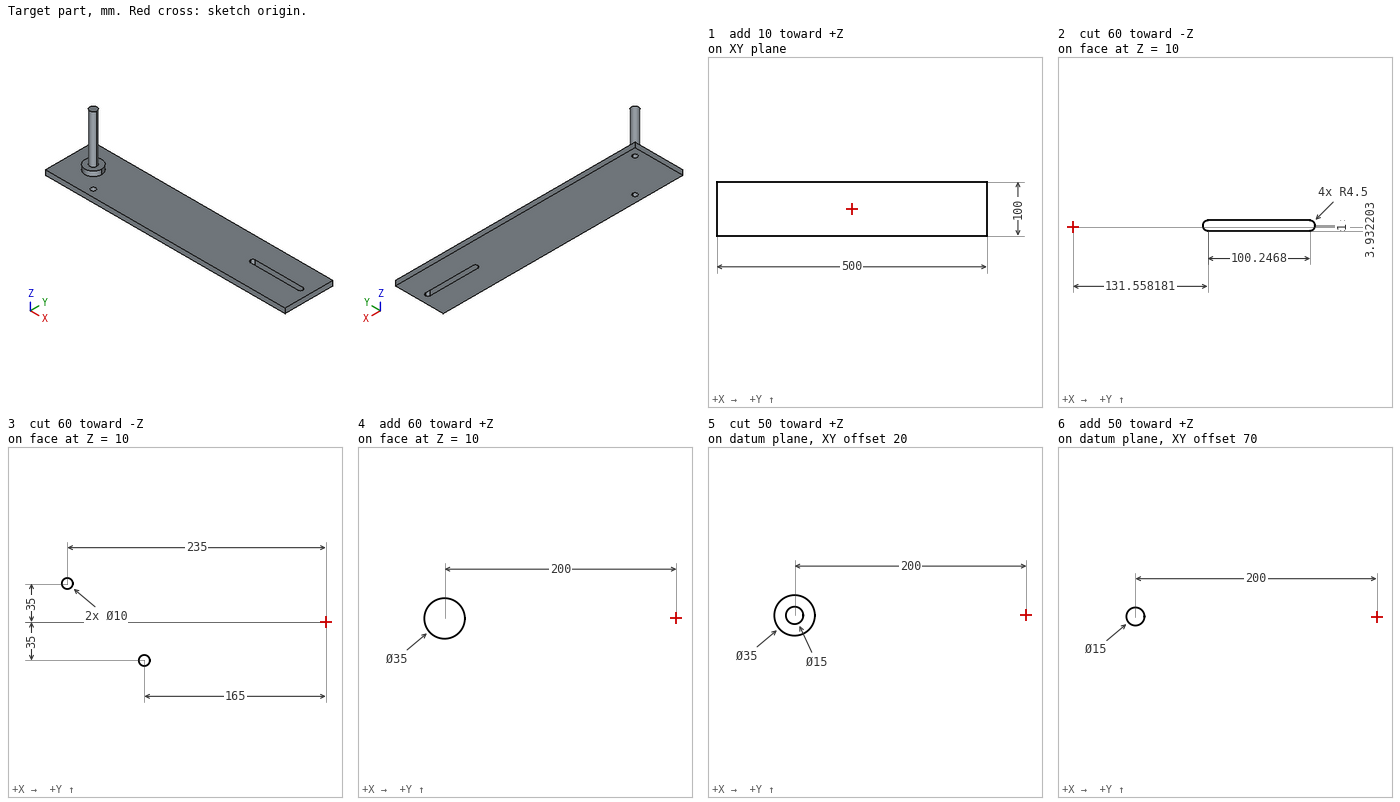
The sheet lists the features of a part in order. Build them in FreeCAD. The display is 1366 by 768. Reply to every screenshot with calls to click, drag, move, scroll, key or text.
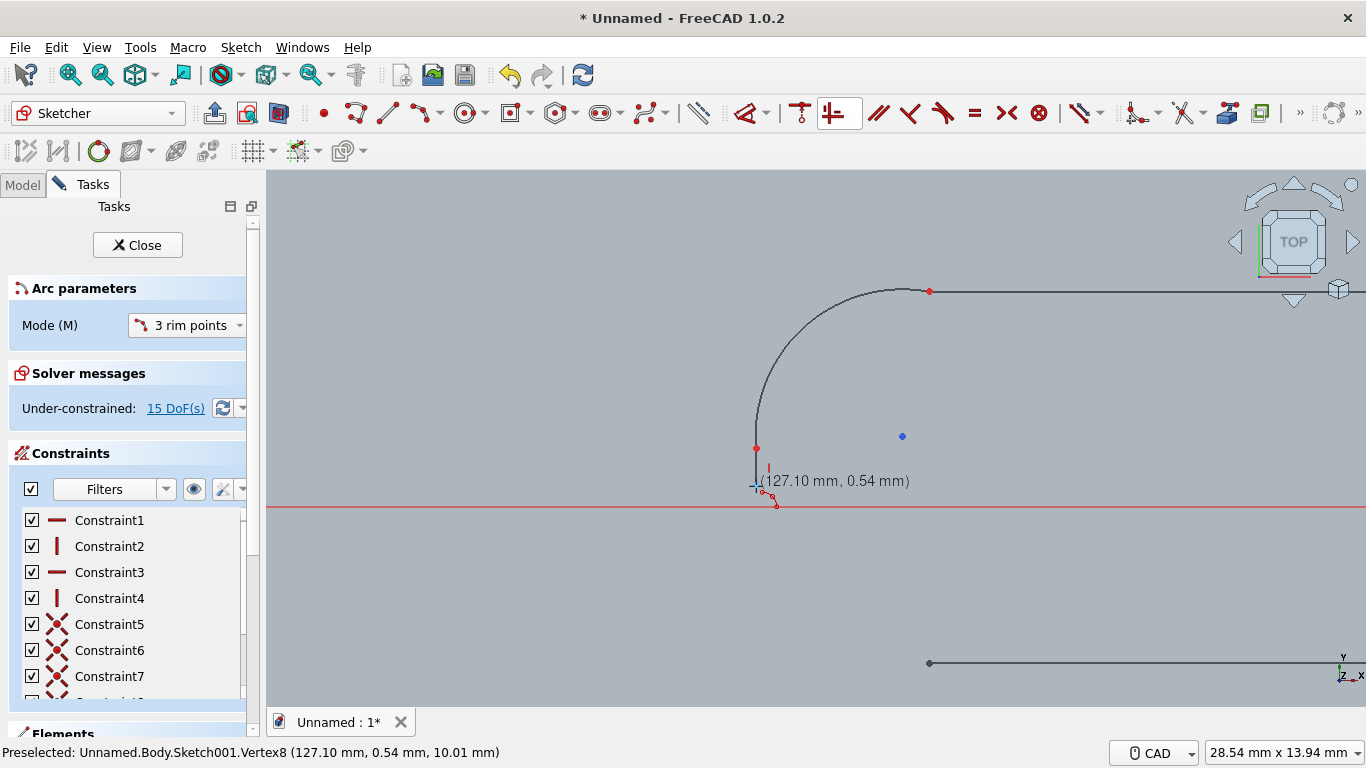
scroll(774, 436, down, 13)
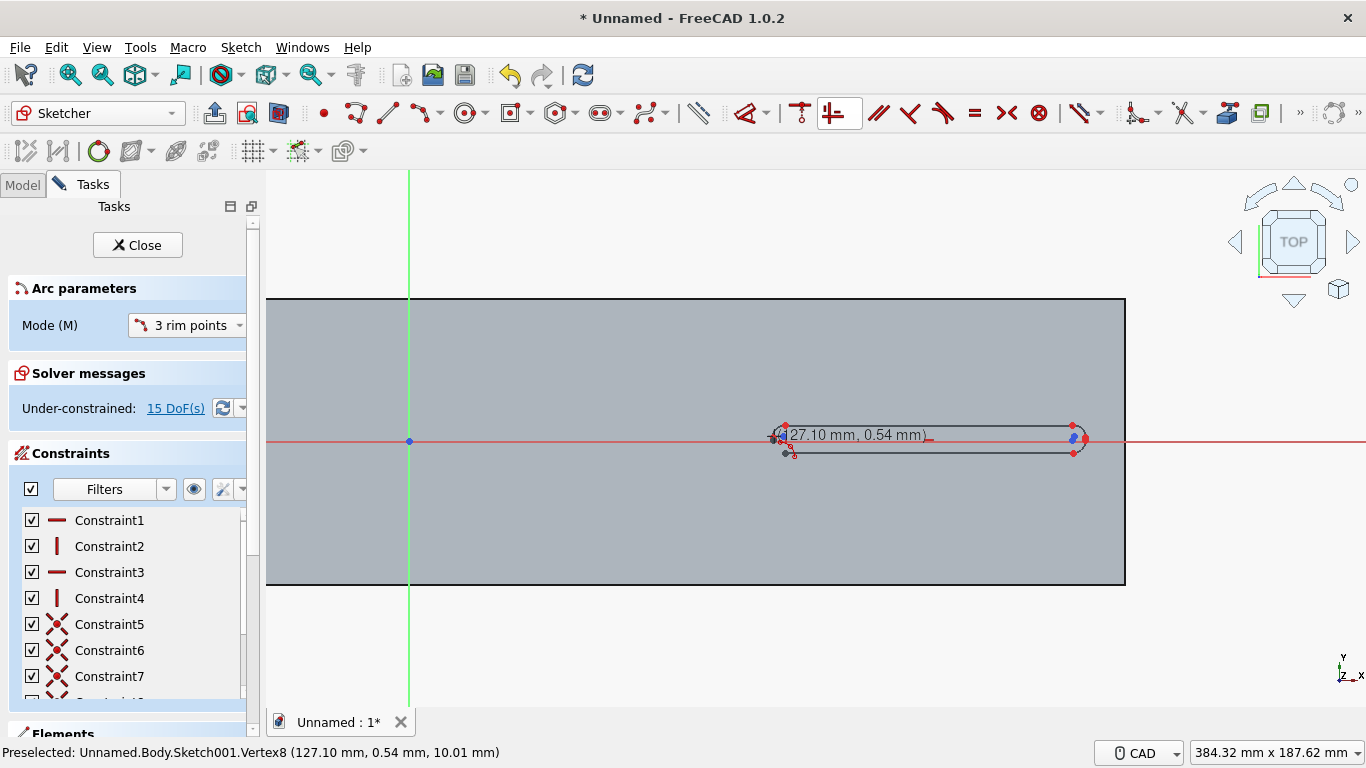
scroll(786, 453, up, 2)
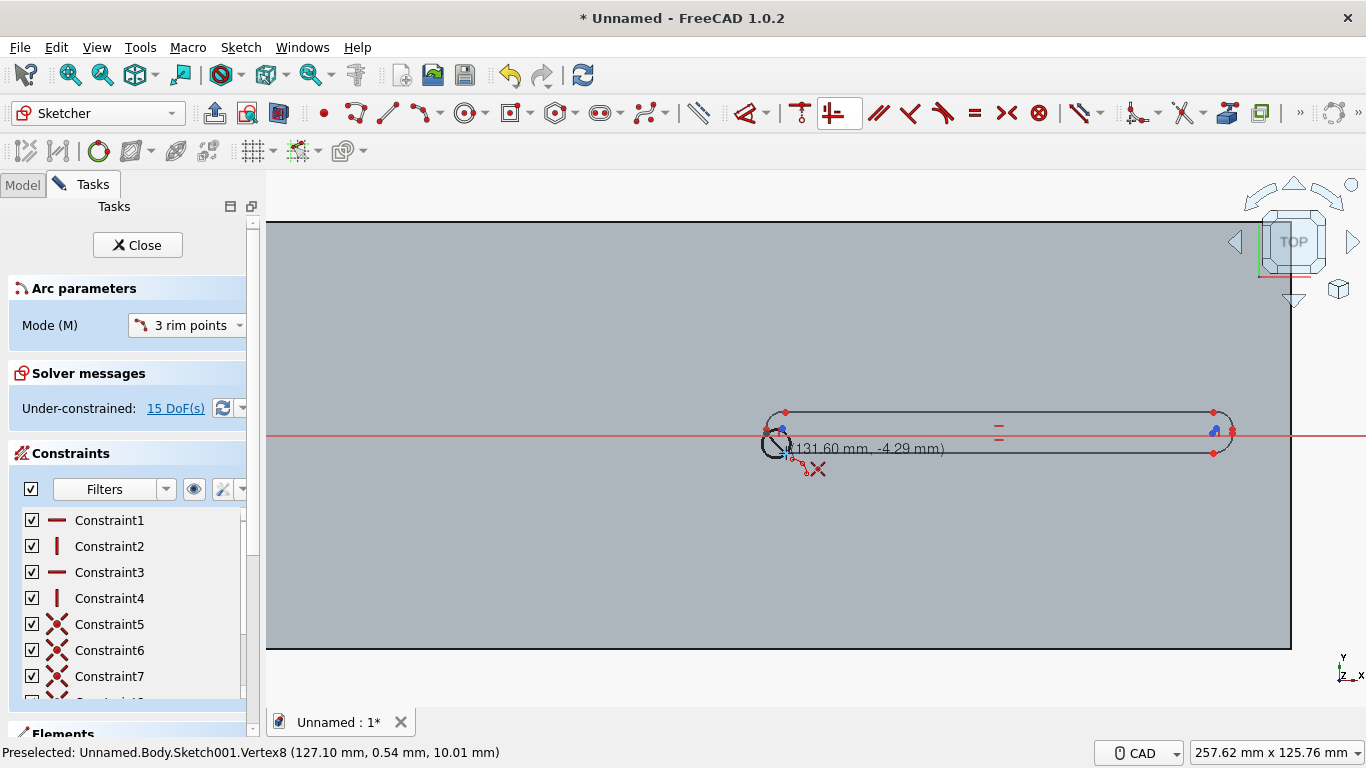
click(786, 453)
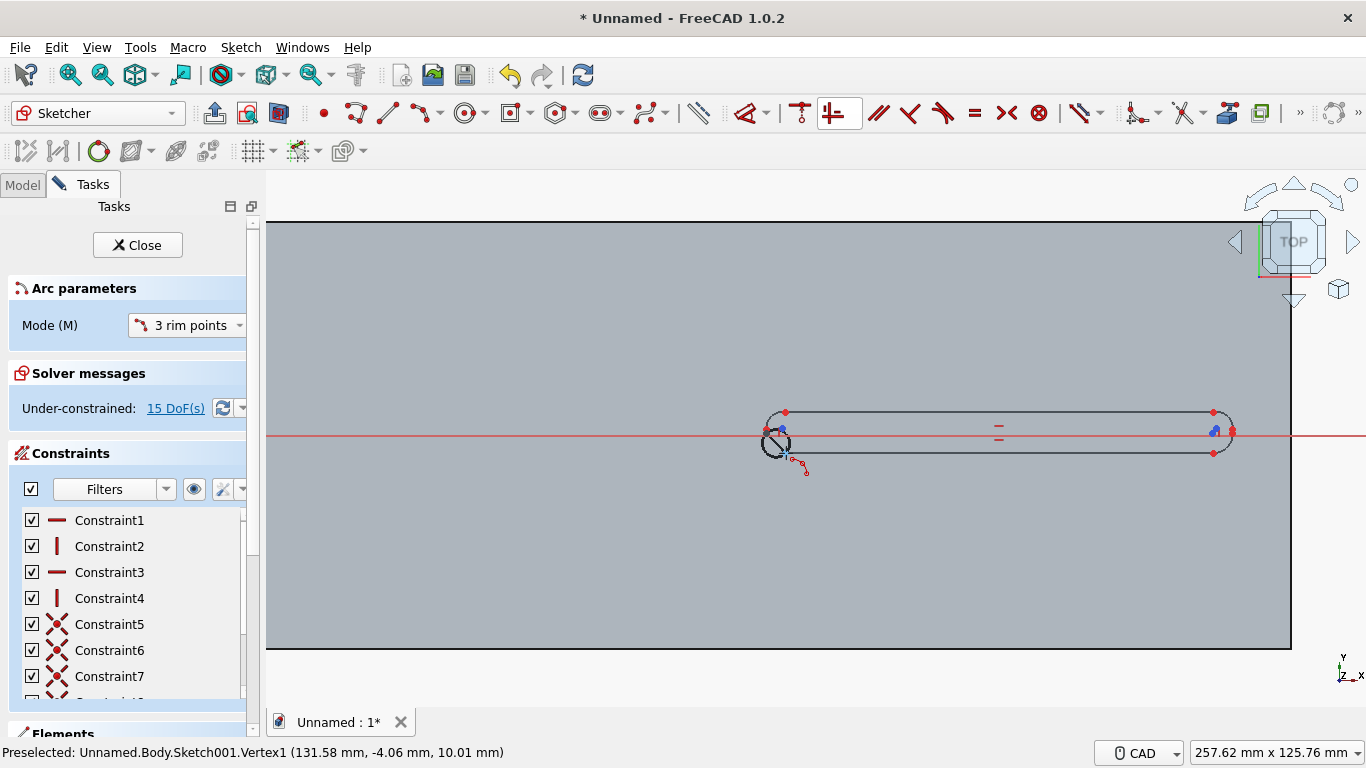
scroll(772, 447, up, 6)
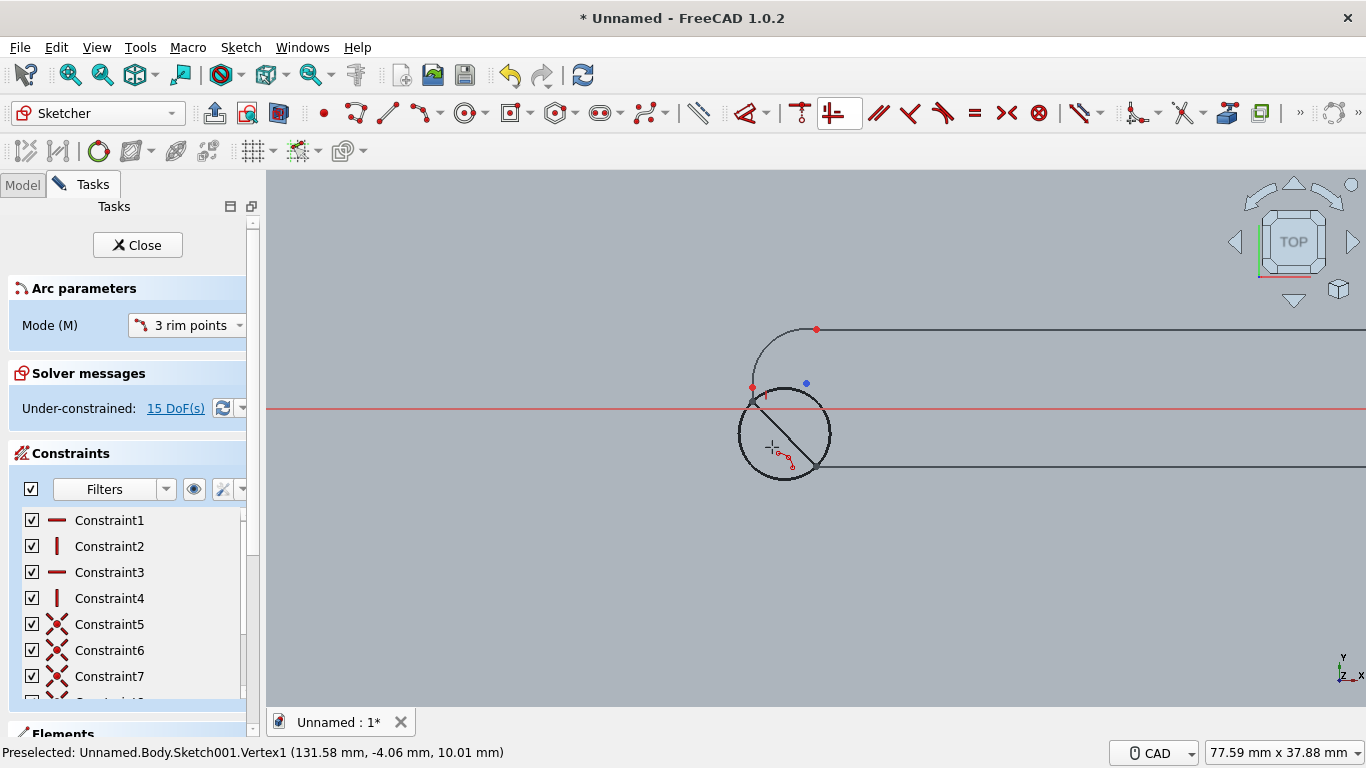
click(771, 446)
key(Escape)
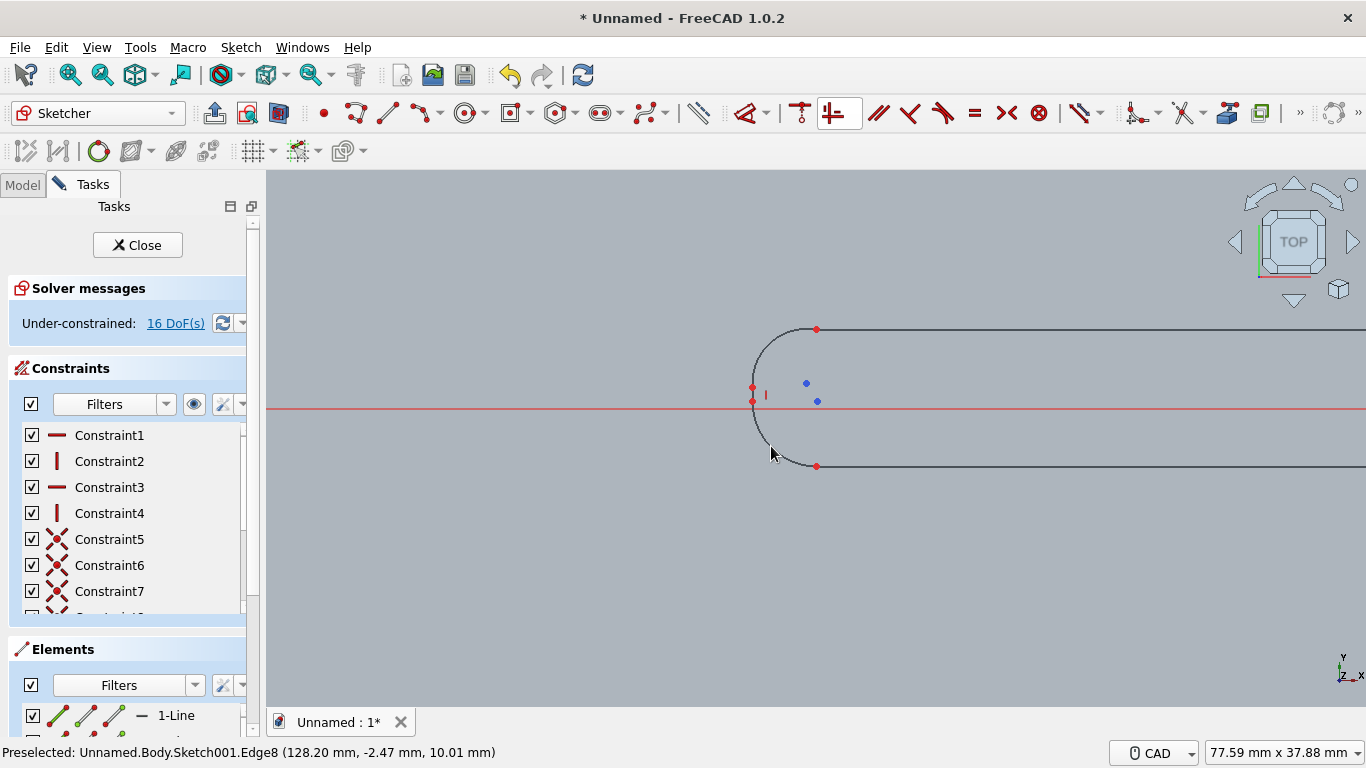
scroll(778, 450, down, 8)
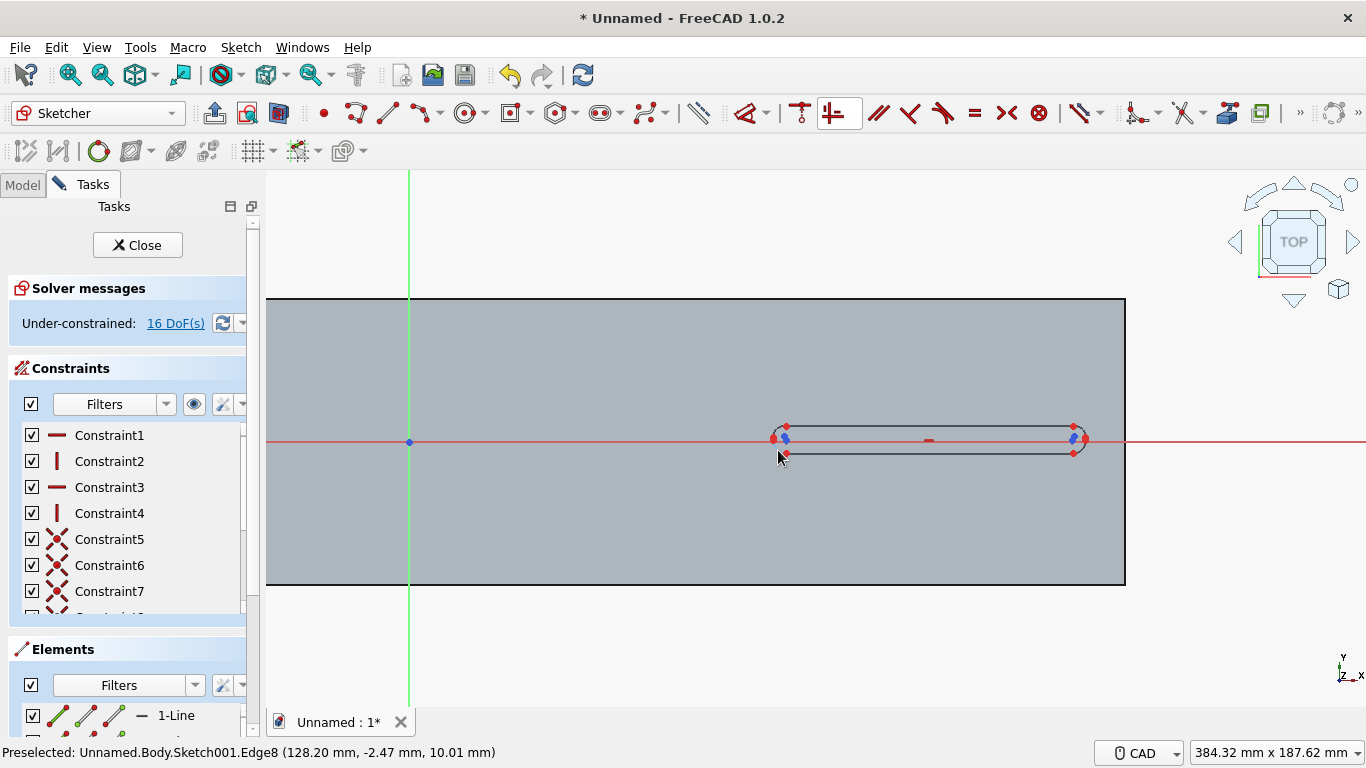
click(844, 454)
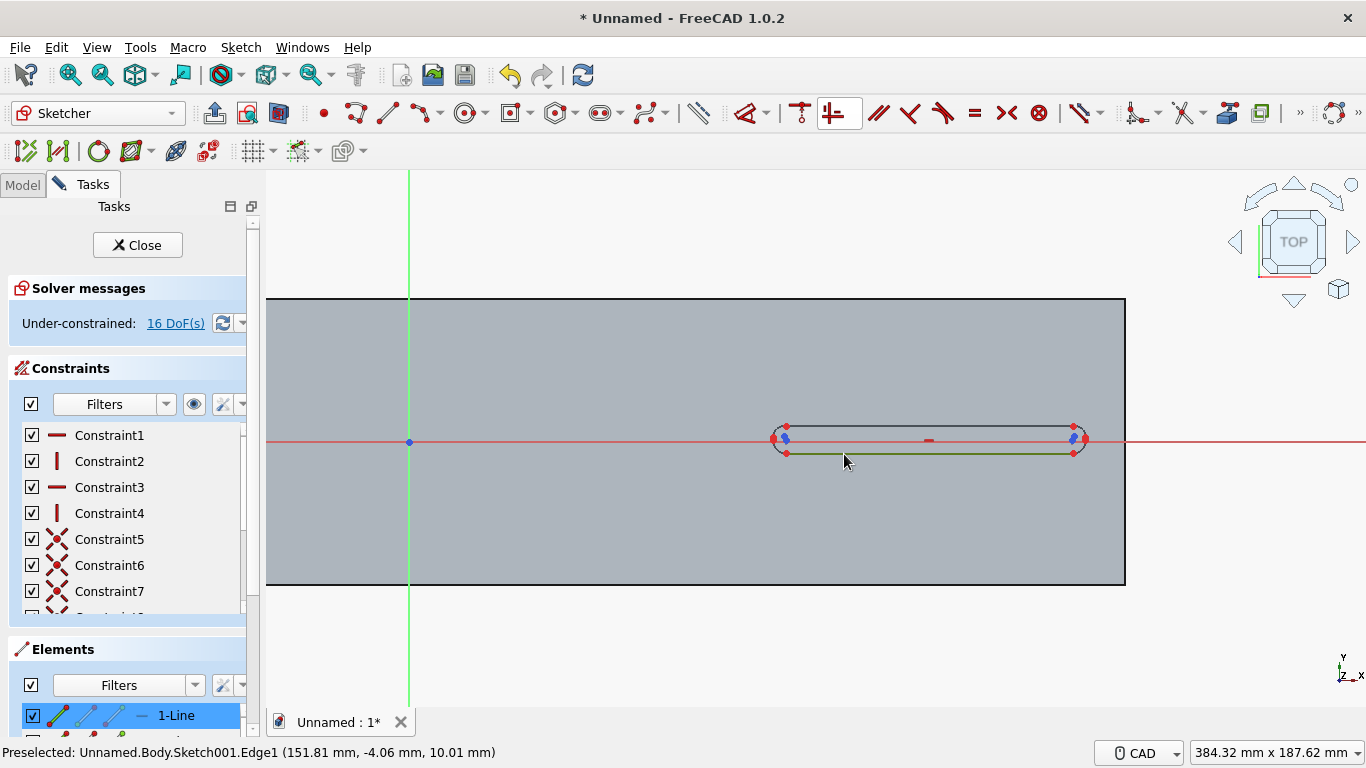
scroll(1082, 450, up, 4)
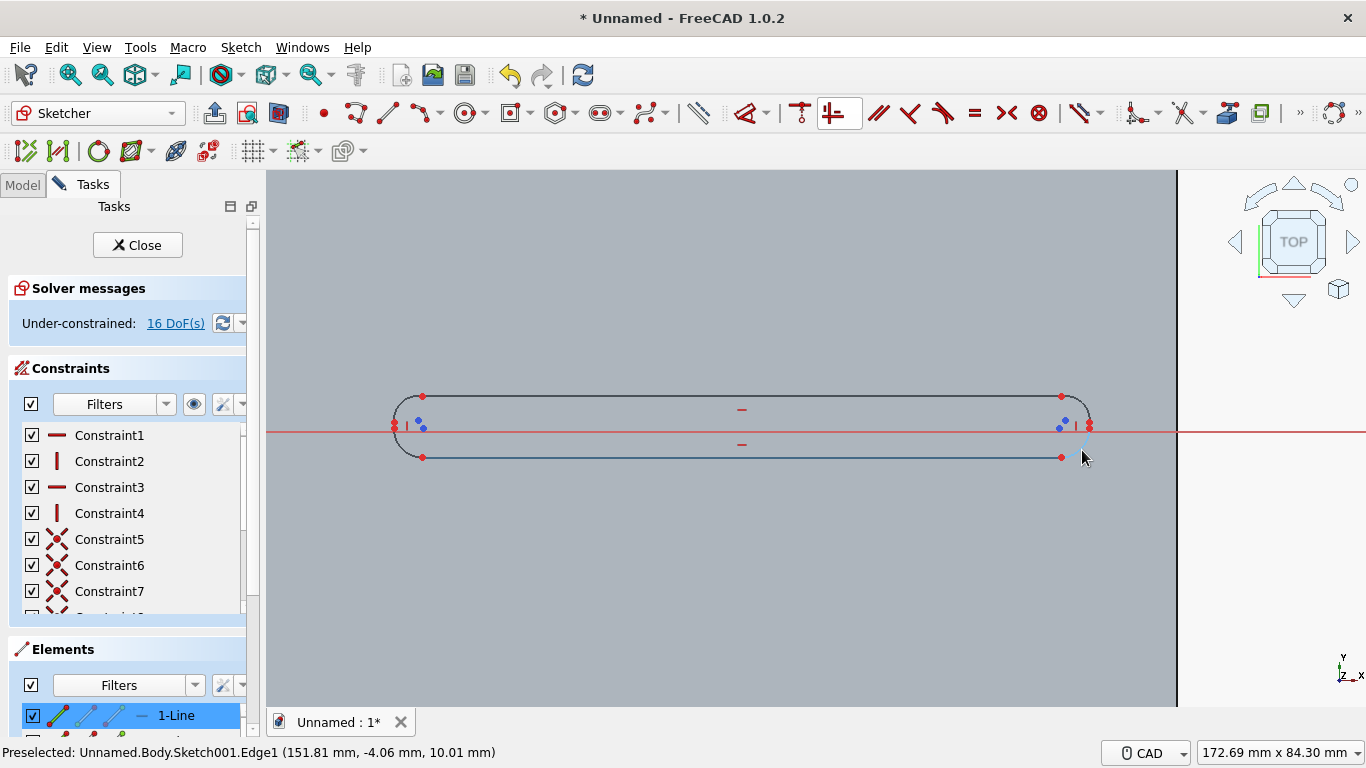
click(1081, 449)